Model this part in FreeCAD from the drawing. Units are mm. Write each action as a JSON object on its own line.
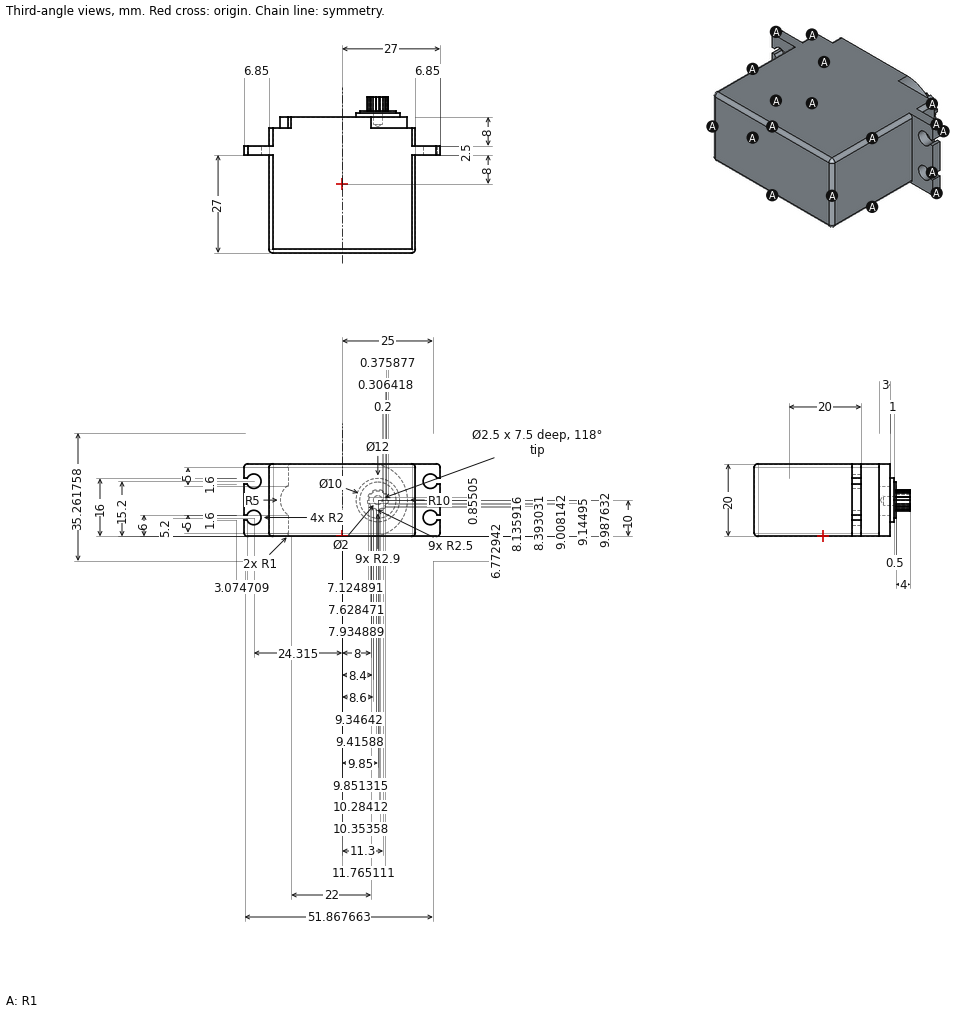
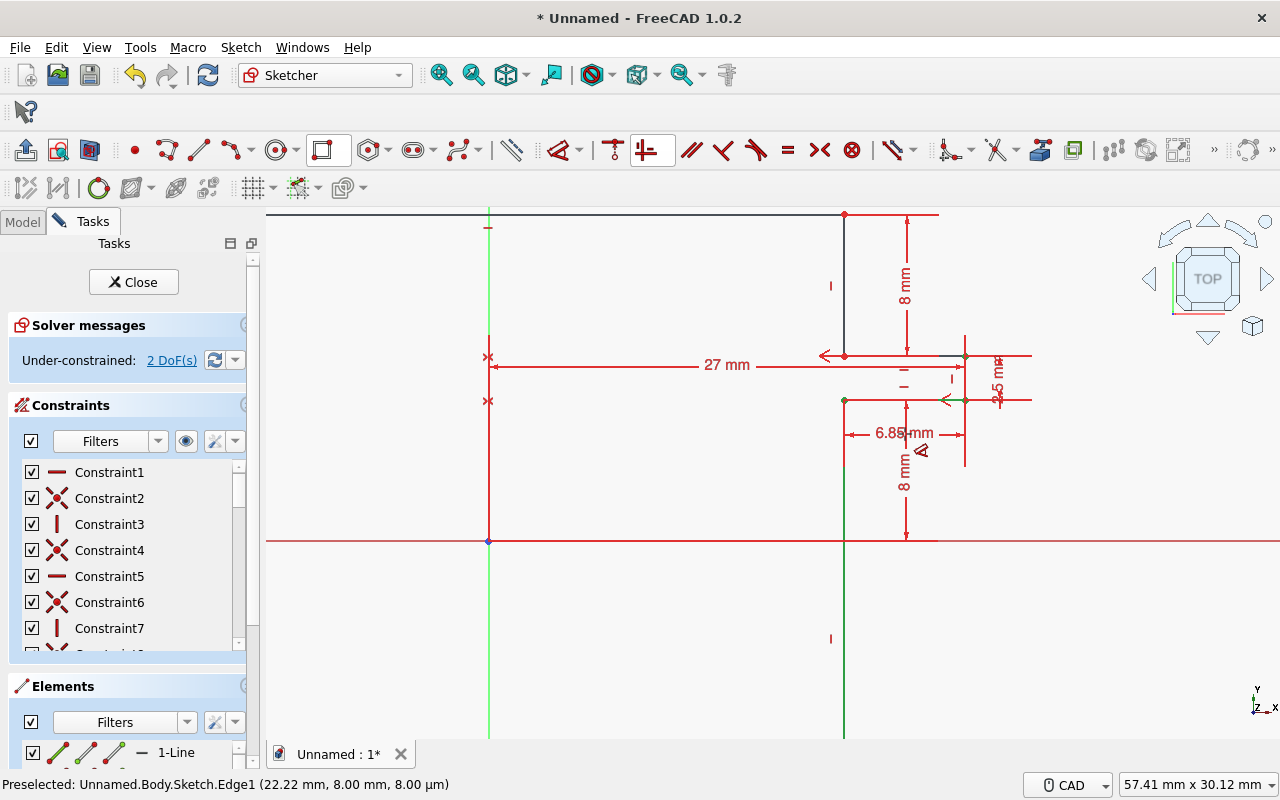
{"action": "left_click", "coordinate": [929, 356]}
{"action": "left_click", "coordinate": [905, 322]}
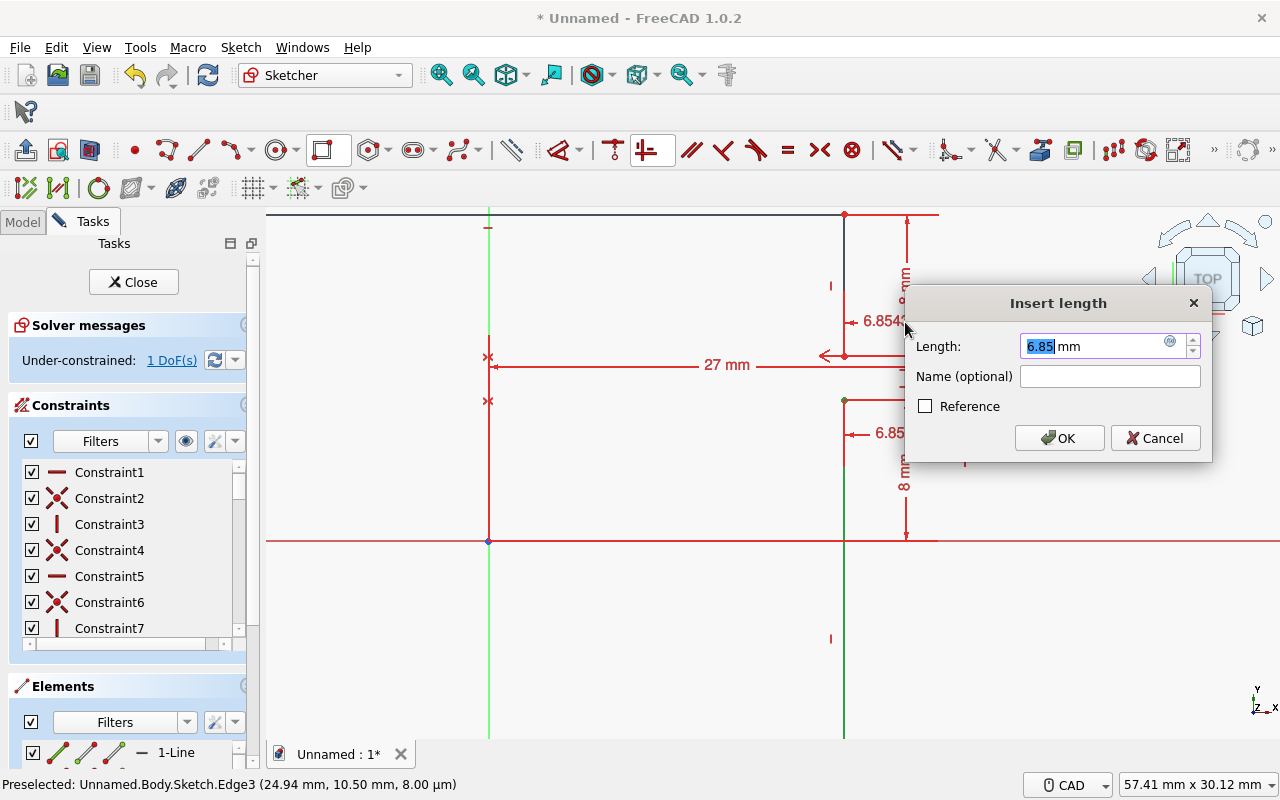
{"action": "type", "text": "6.85"}
{"action": "key", "text": "Return"}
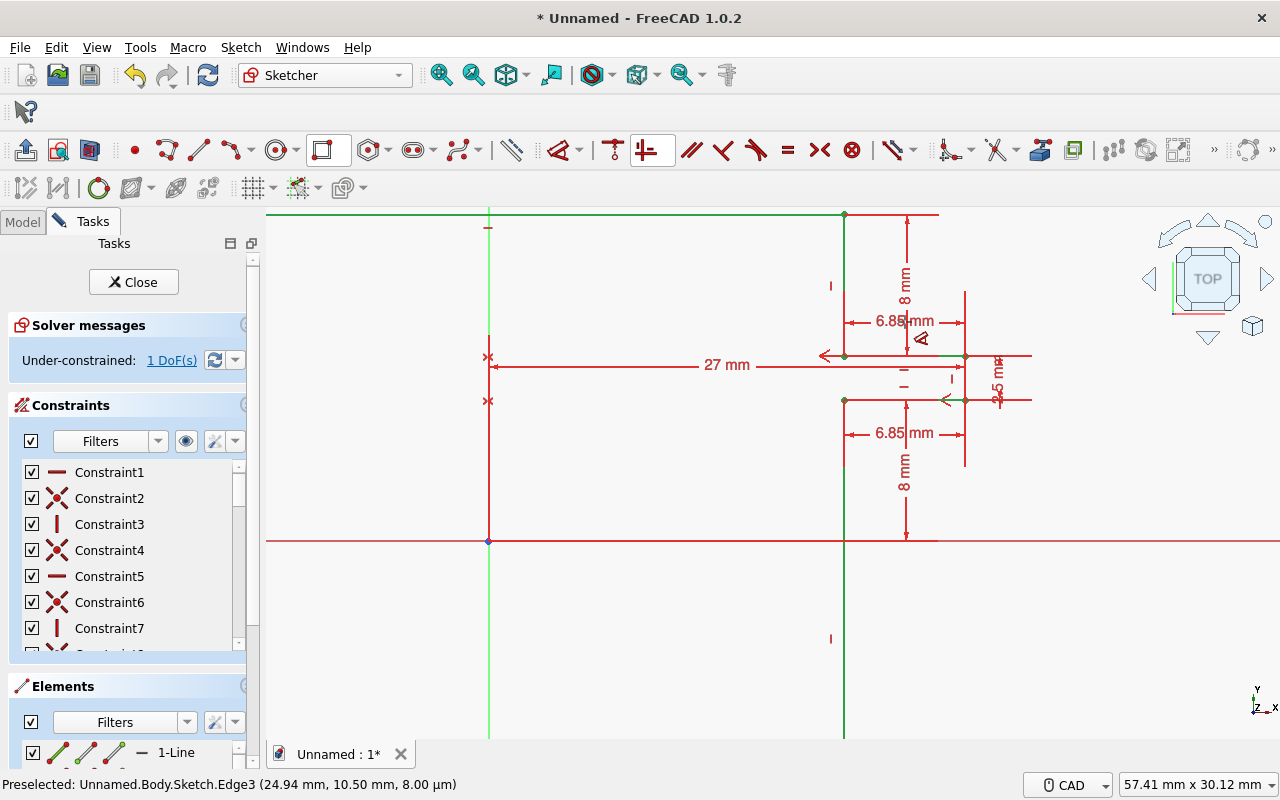
{"action": "scroll", "coordinate": [967, 384], "scroll_direction": "down", "scroll_amount": 3}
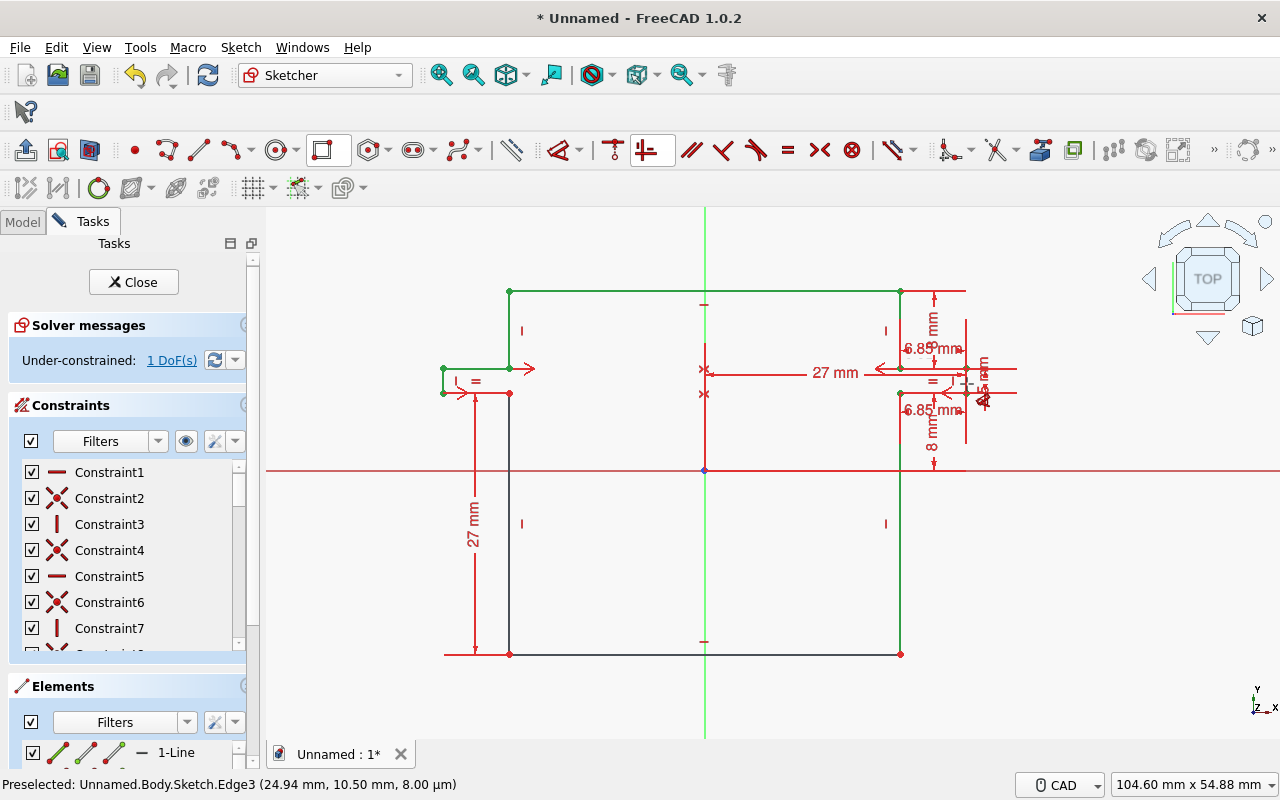
{"action": "left_click", "coordinate": [463, 393]}
{"action": "left_click", "coordinate": [476, 427]}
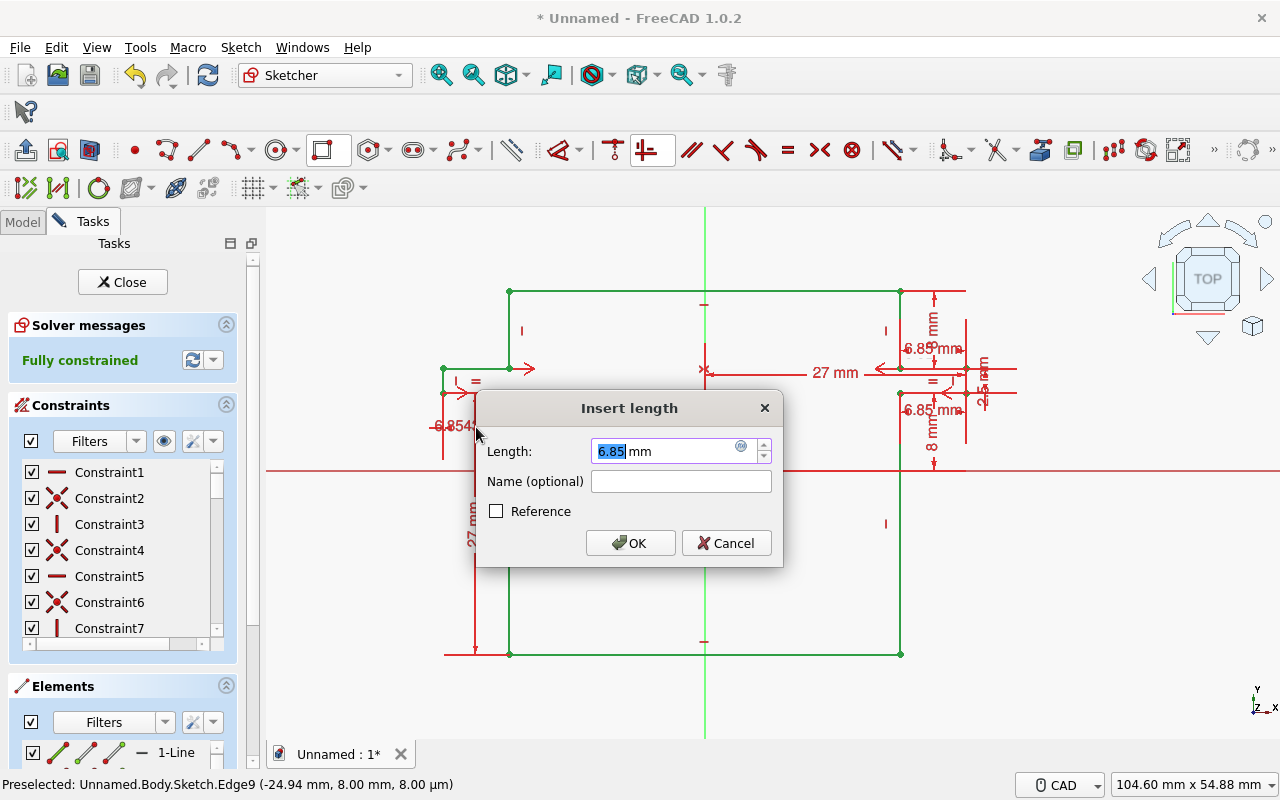
{"action": "type", "text": "6.85"}
{"action": "key", "text": "Return"}
{"action": "key", "text": "Escape"}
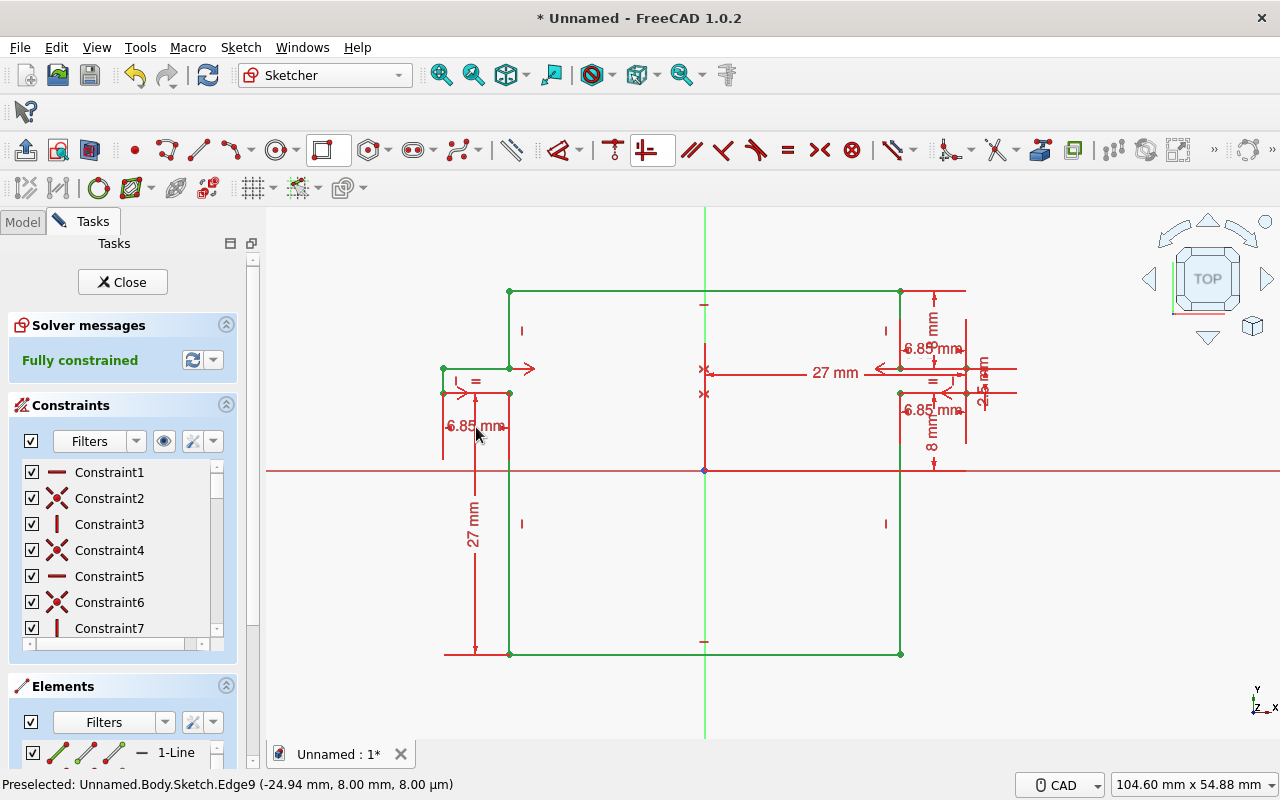
{"action": "left_click", "coordinate": [123, 282]}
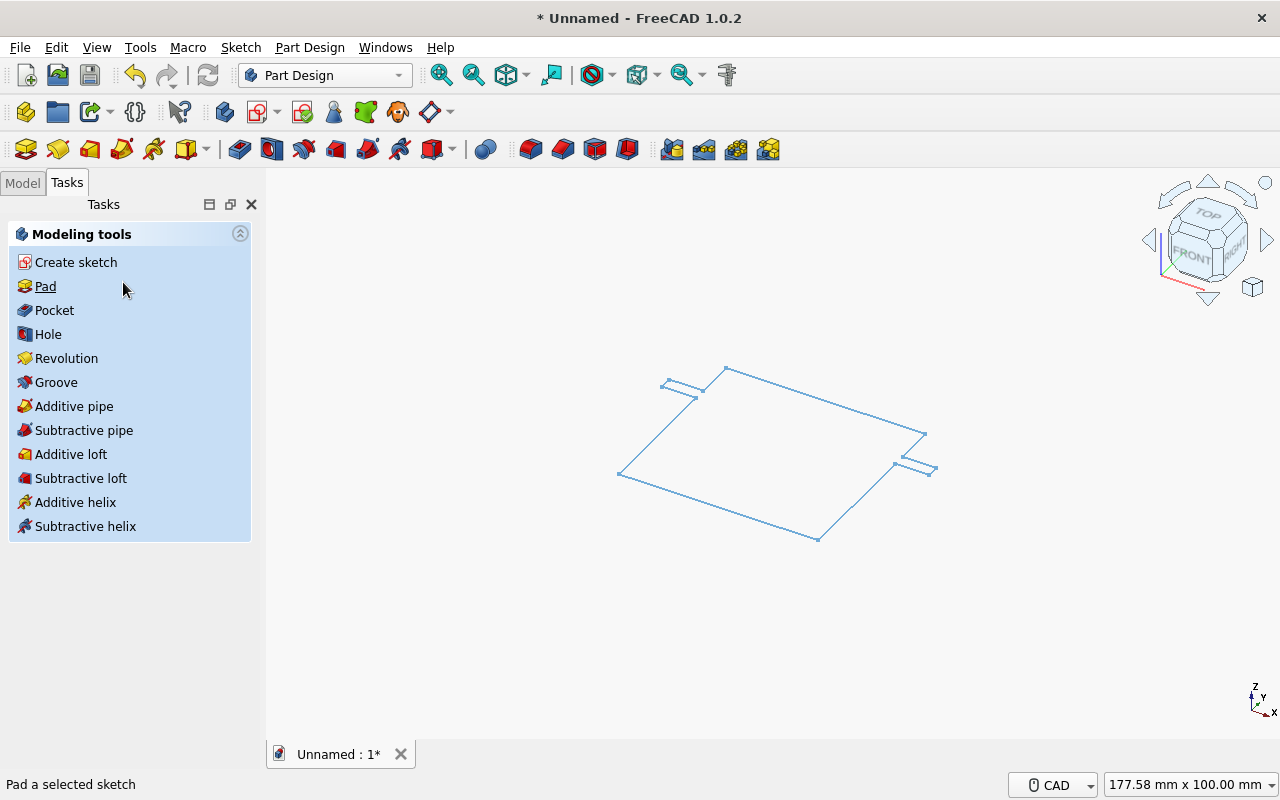
{"action": "left_click", "coordinate": [26, 150]}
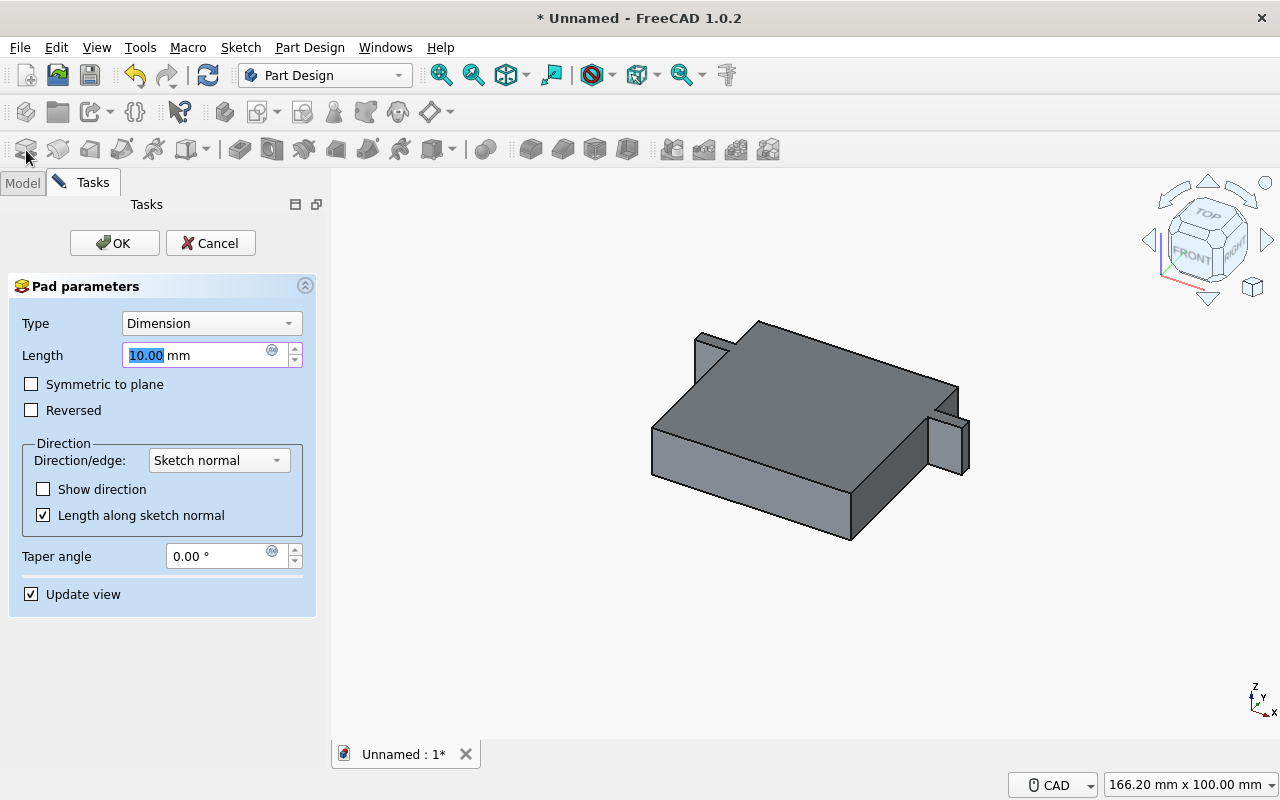
{"action": "type", "text": "20"}
{"action": "key", "text": "Tab"}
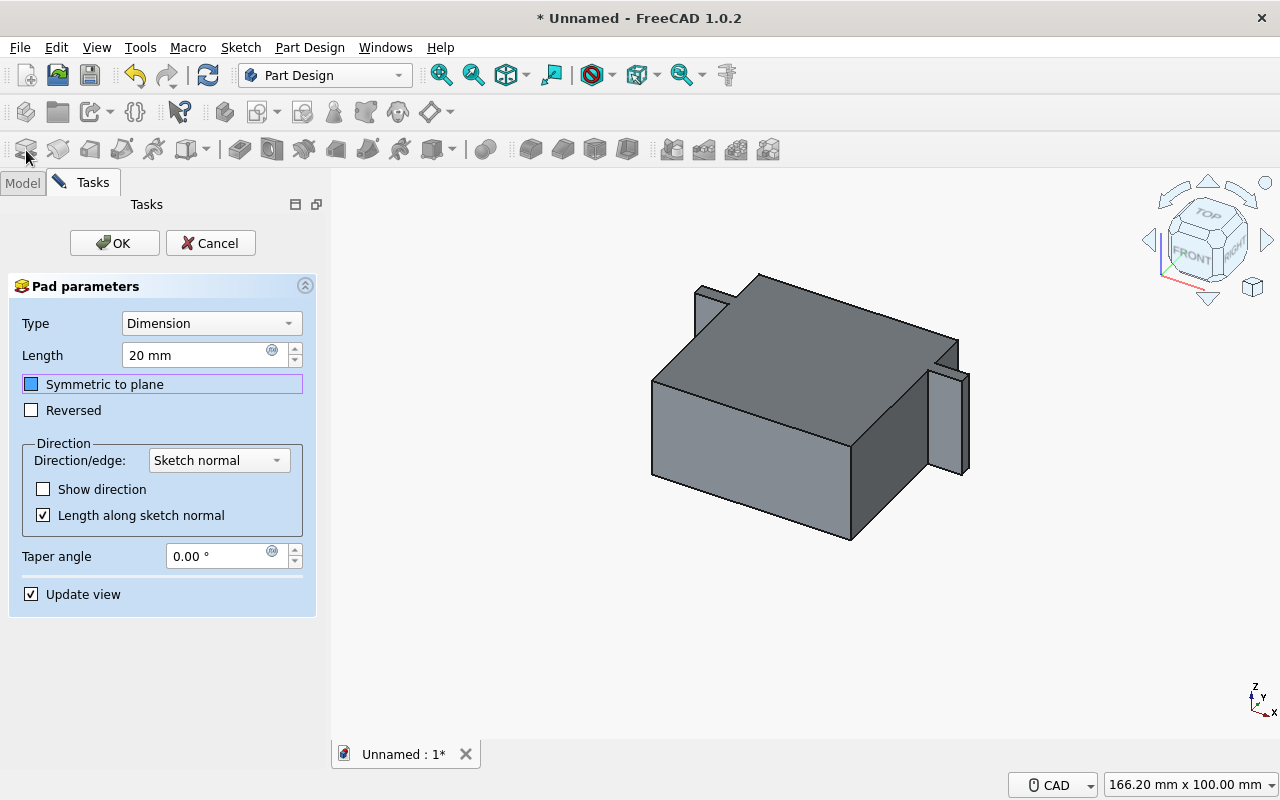
{"action": "left_click", "coordinate": [115, 243]}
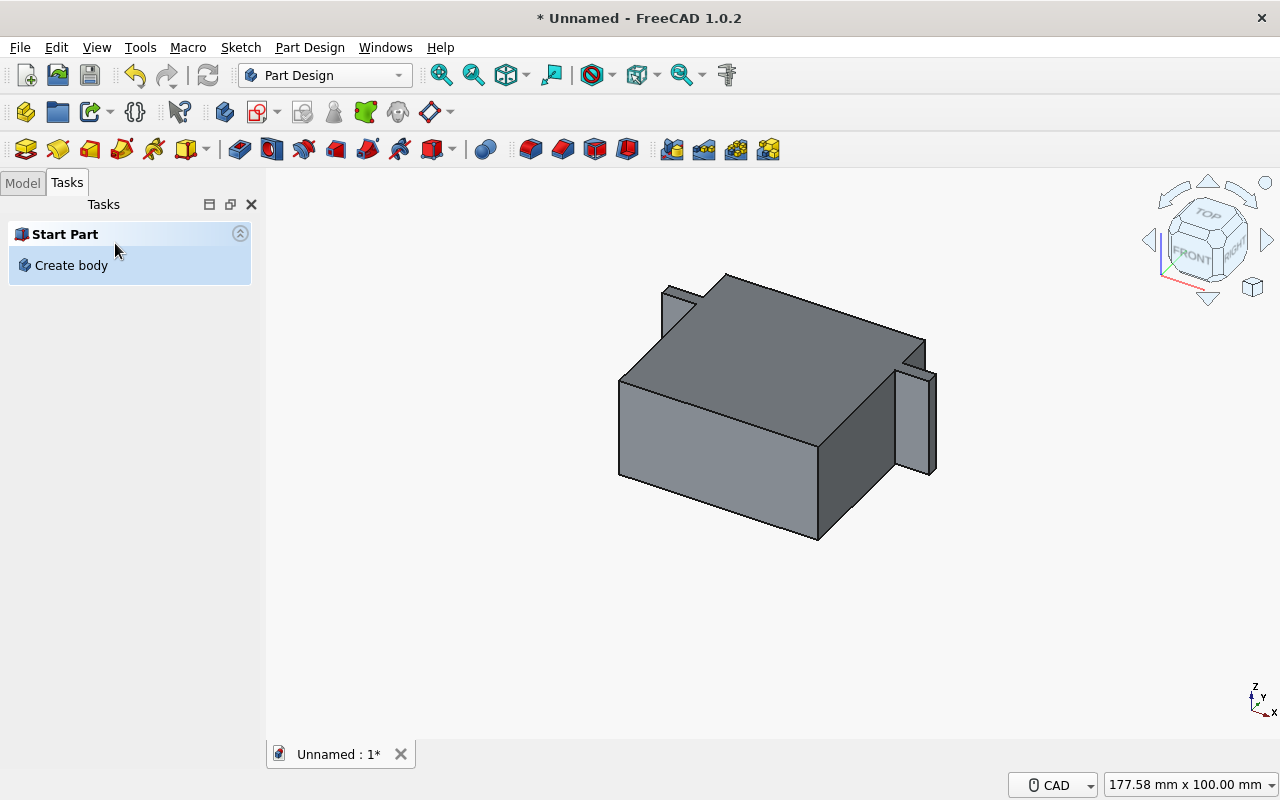
{"action": "left_click", "coordinate": [747, 469]}